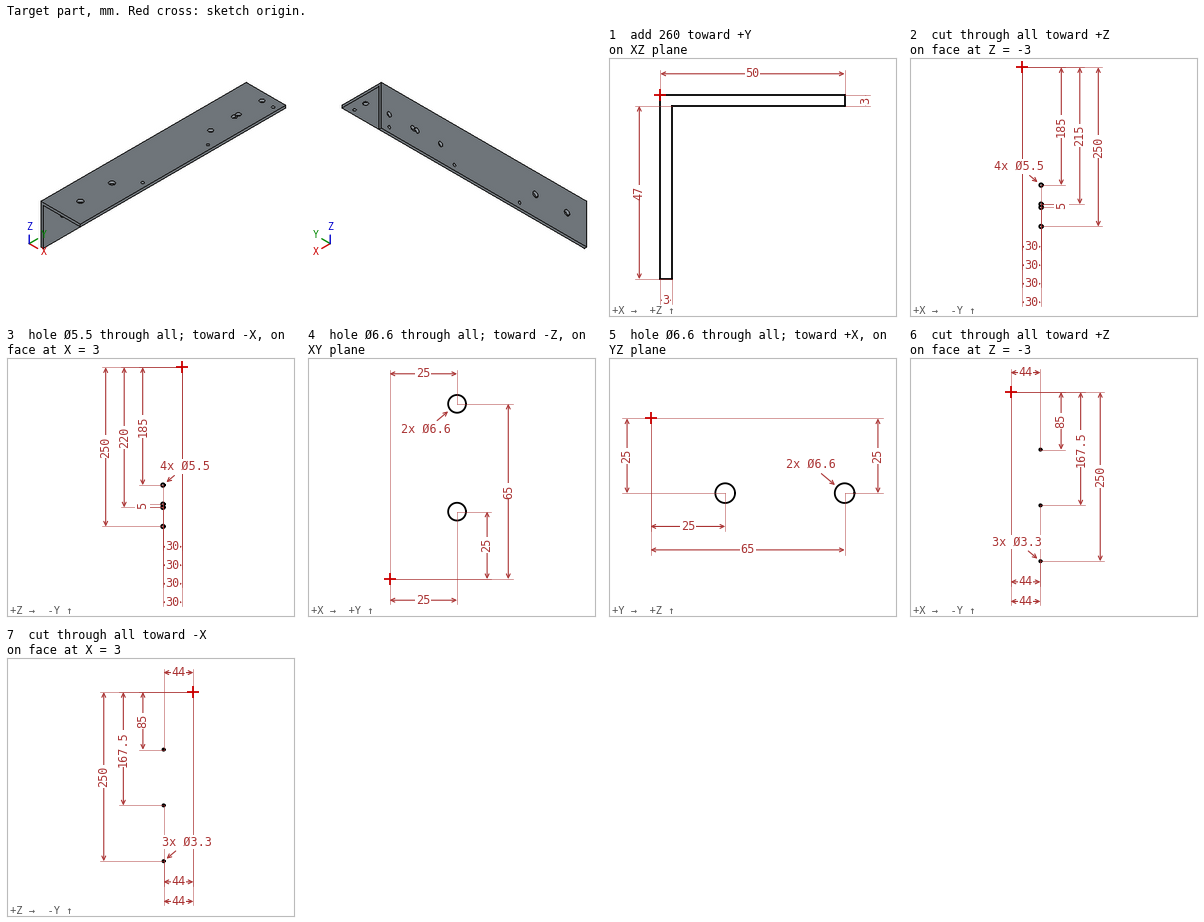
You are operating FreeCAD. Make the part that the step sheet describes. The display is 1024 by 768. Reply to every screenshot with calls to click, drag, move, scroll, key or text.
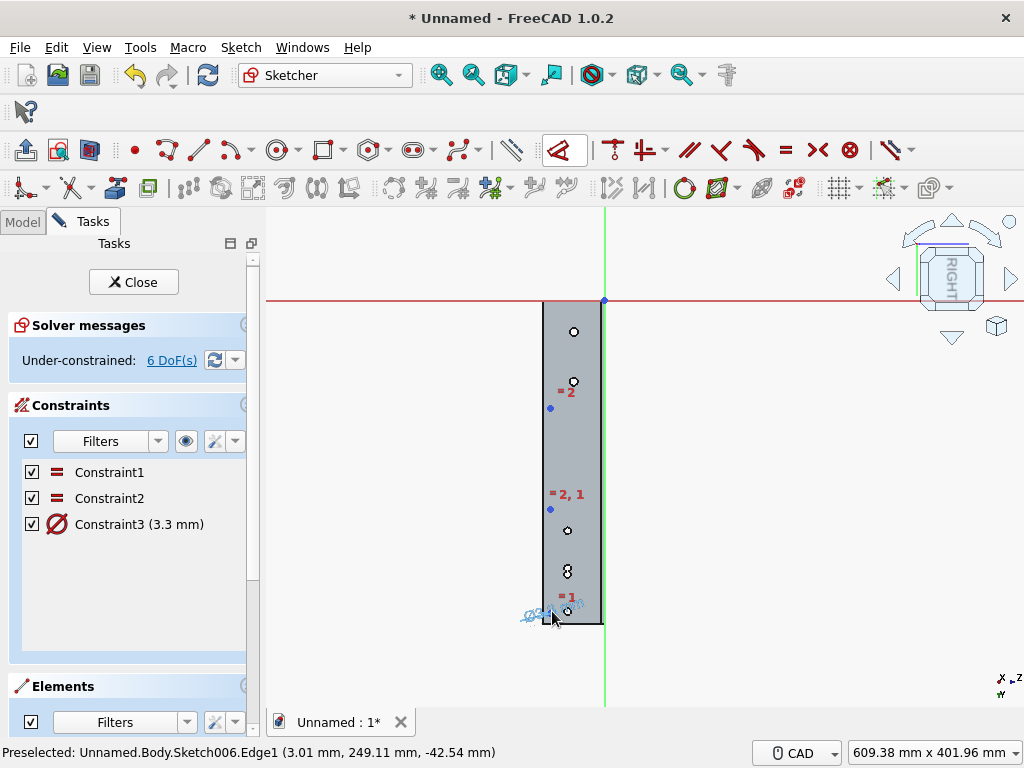
click(550, 613)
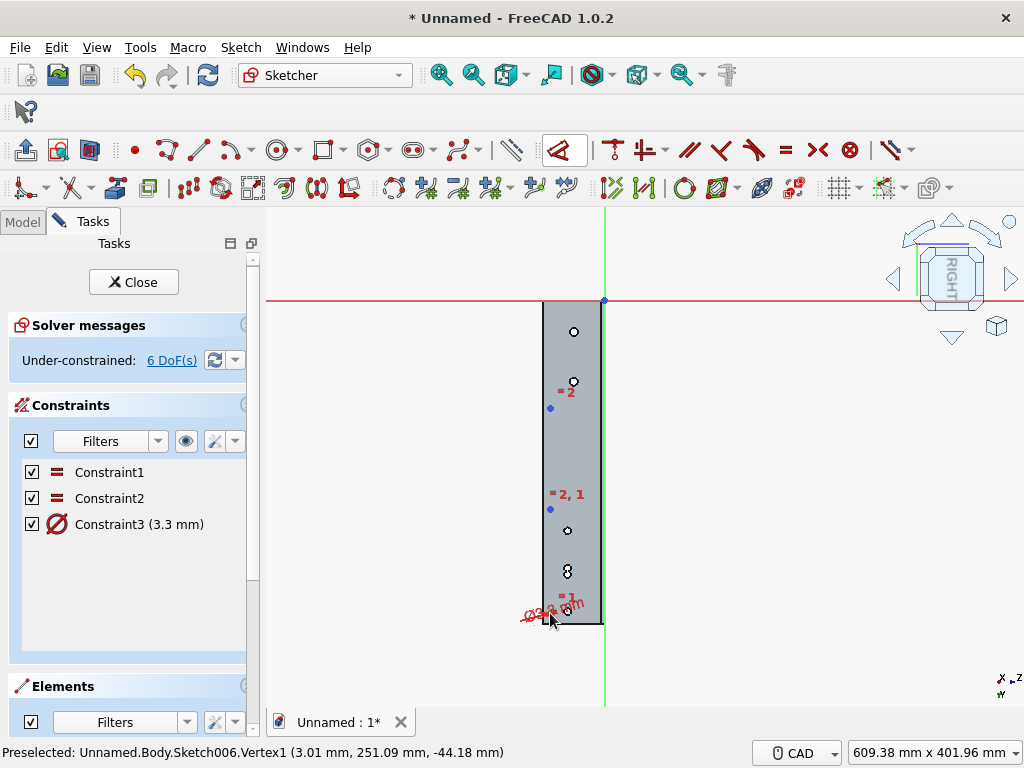
key(l)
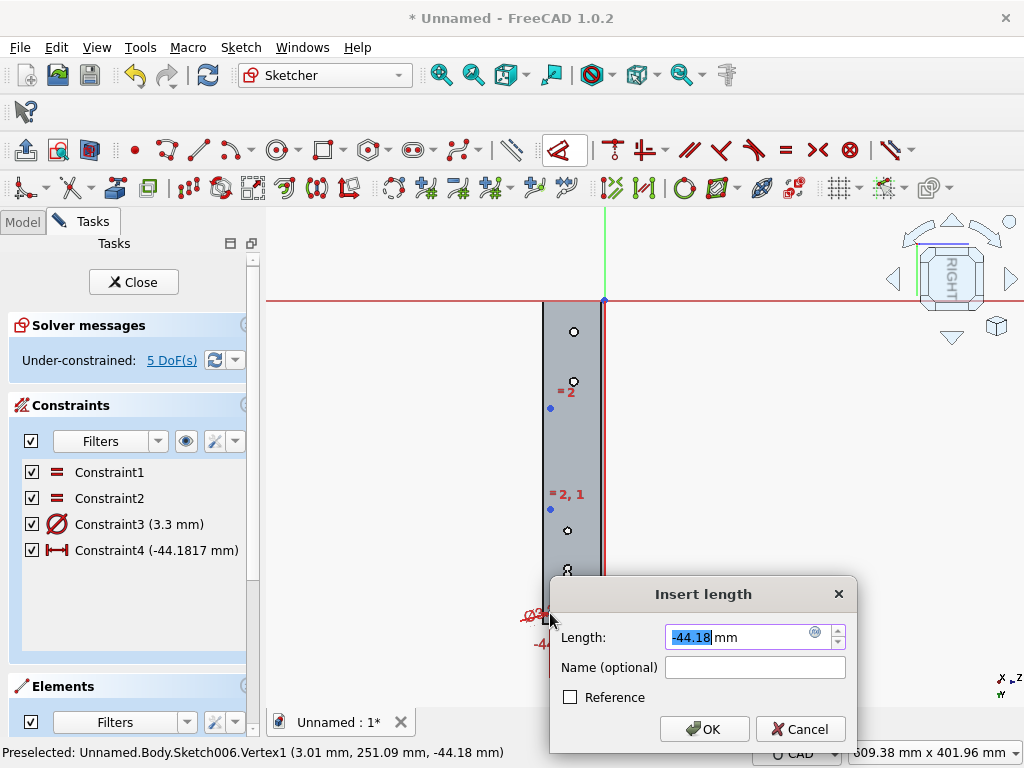
text(-44)
key(Return)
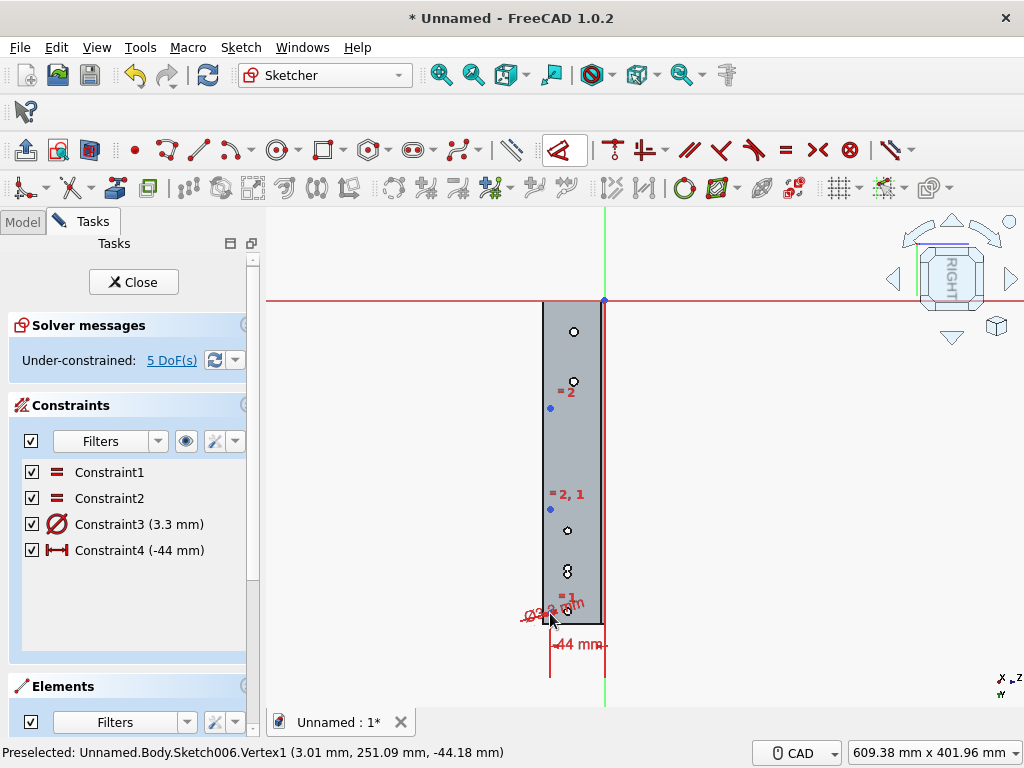
click(550, 510)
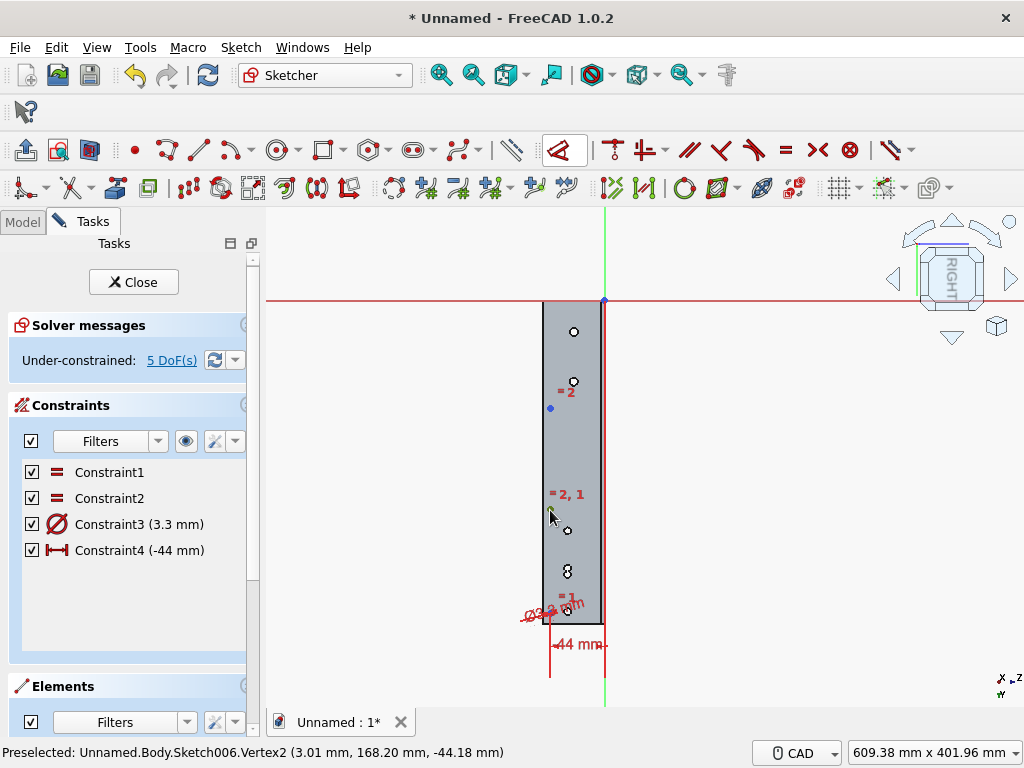
key(l)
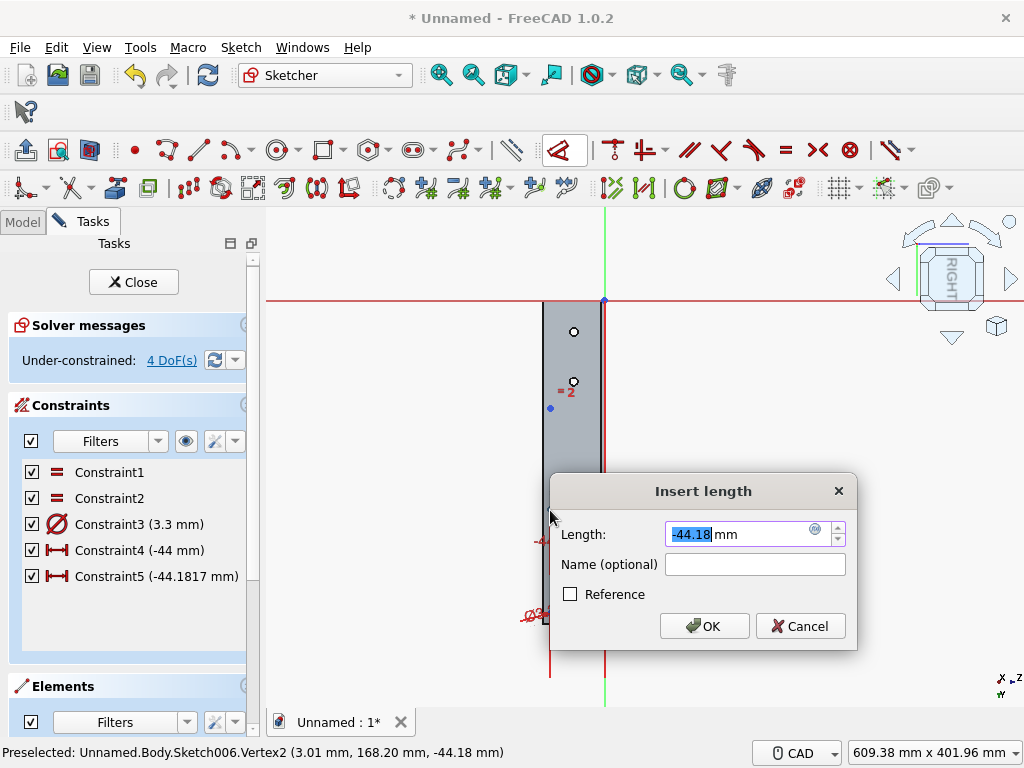
text(-44)
key(Return)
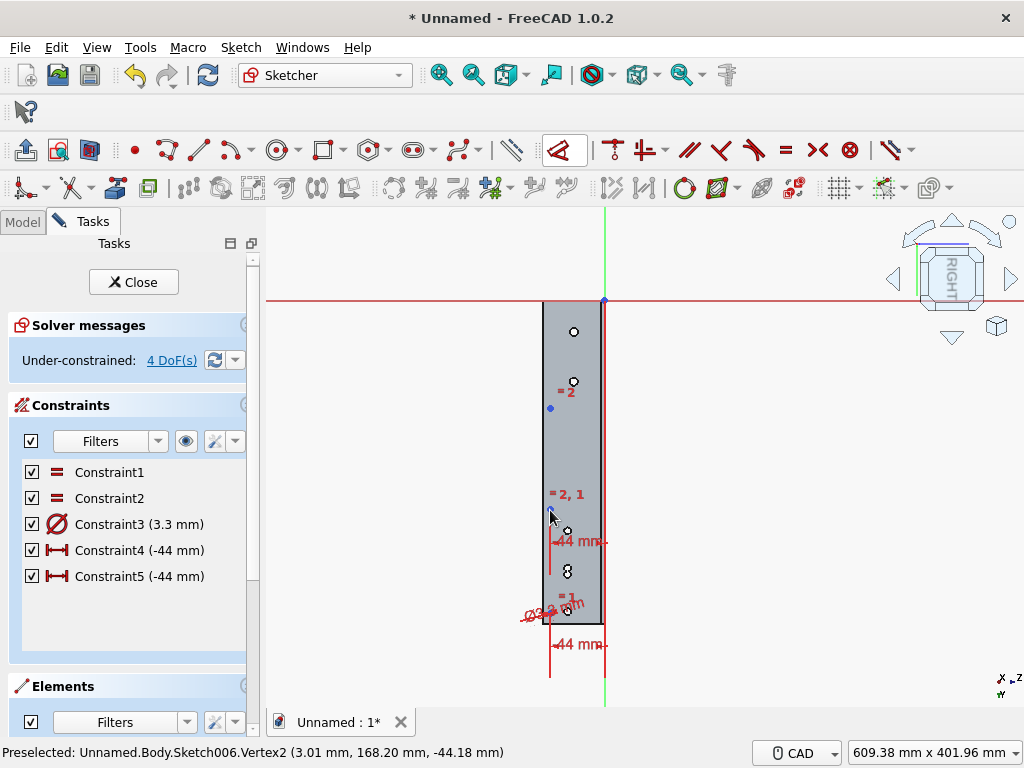
click(550, 408)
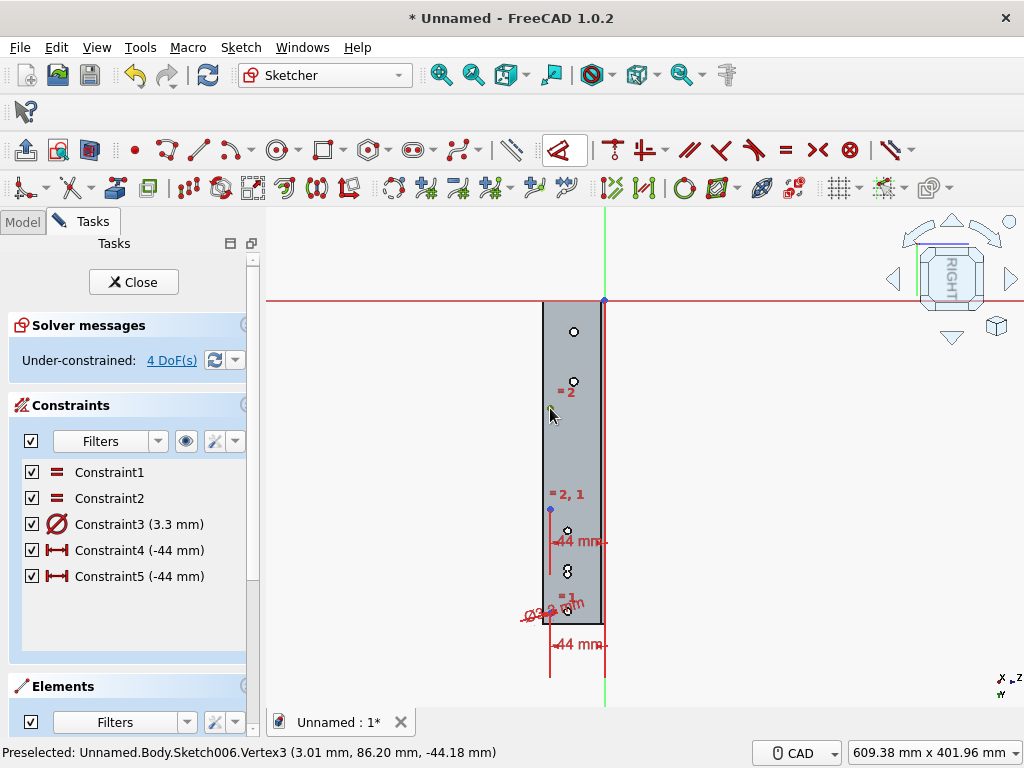
key(l)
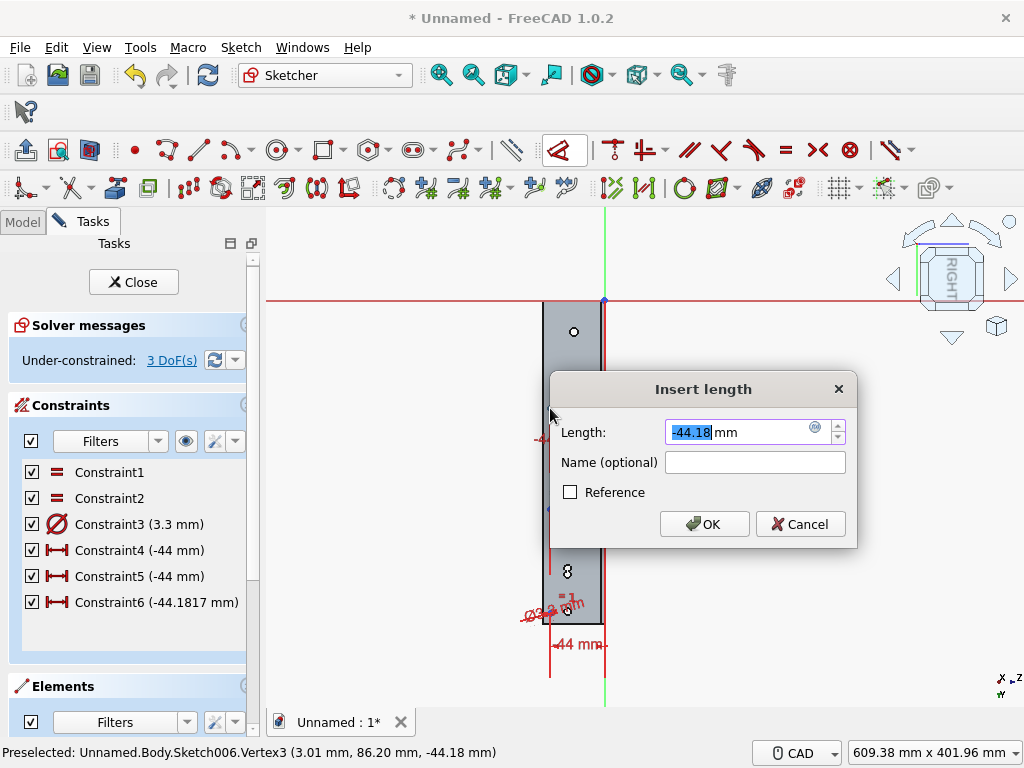
text(-44)
key(Return)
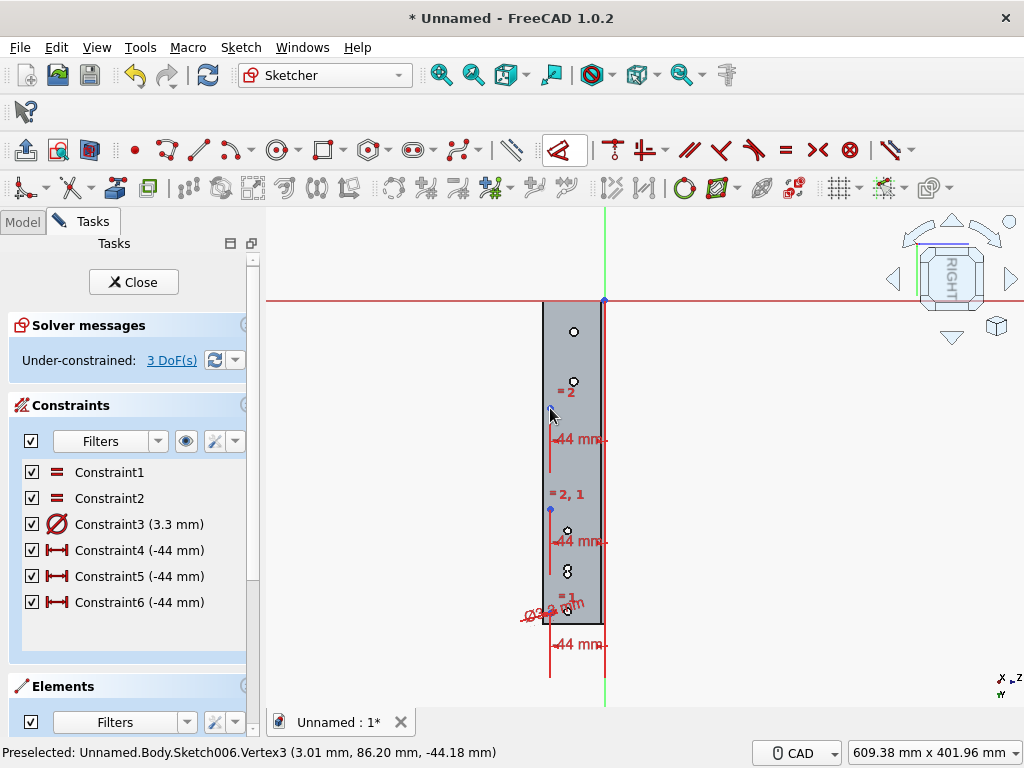
click(550, 408)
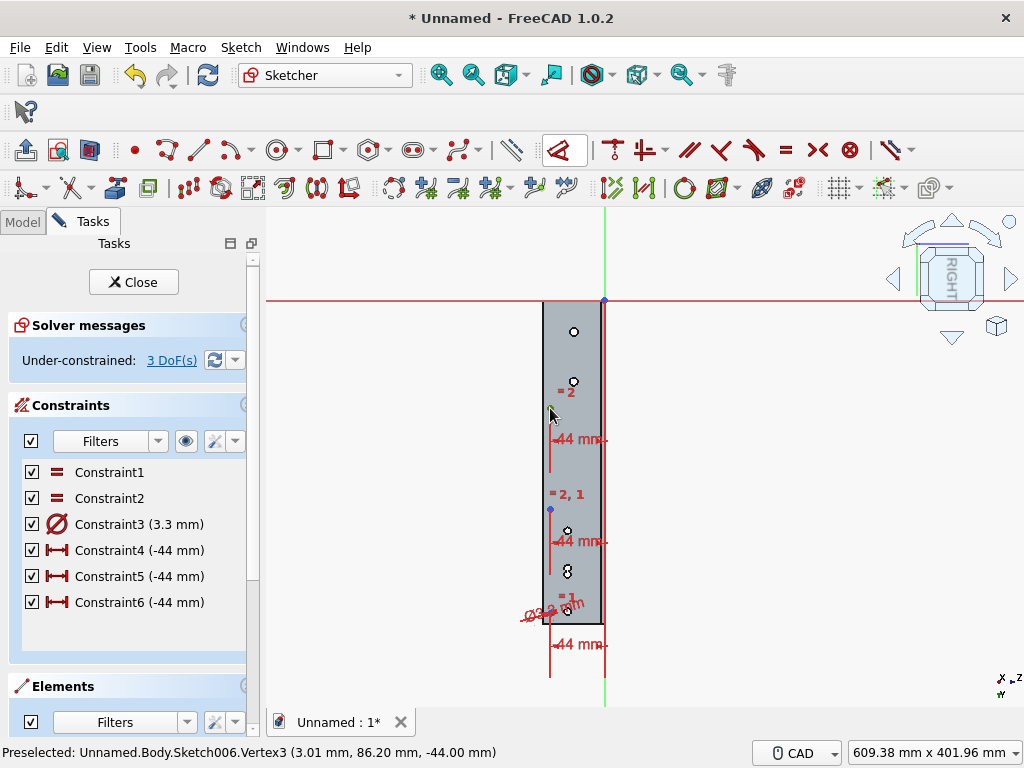
key(i)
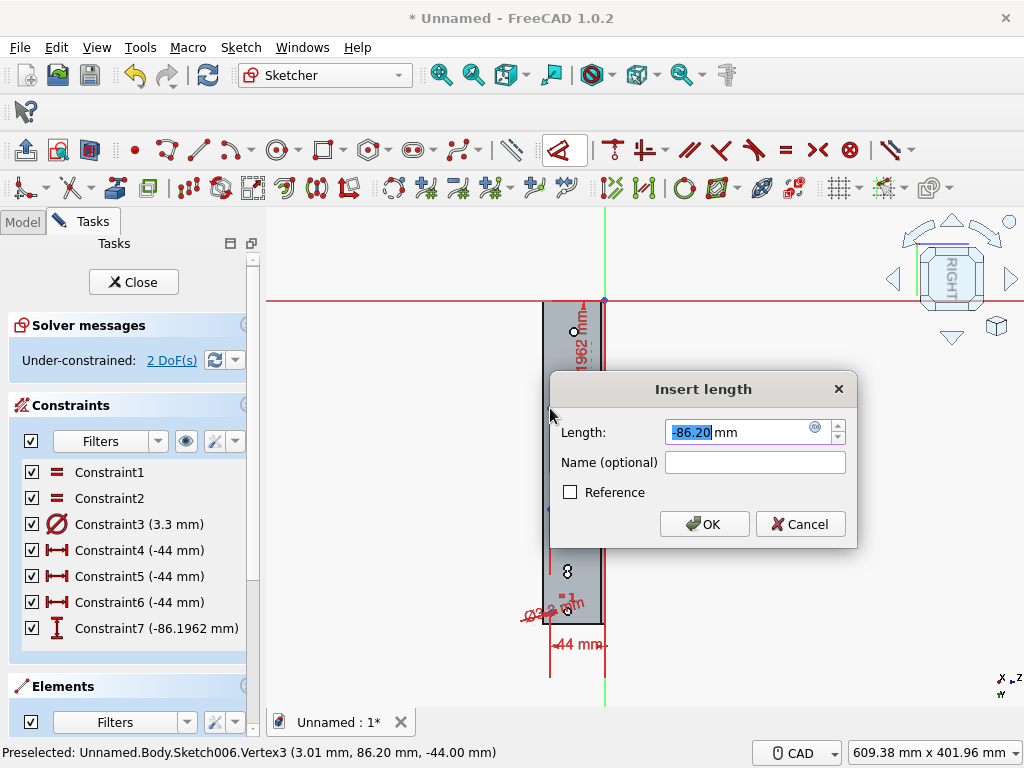
text(-85)
key(Return)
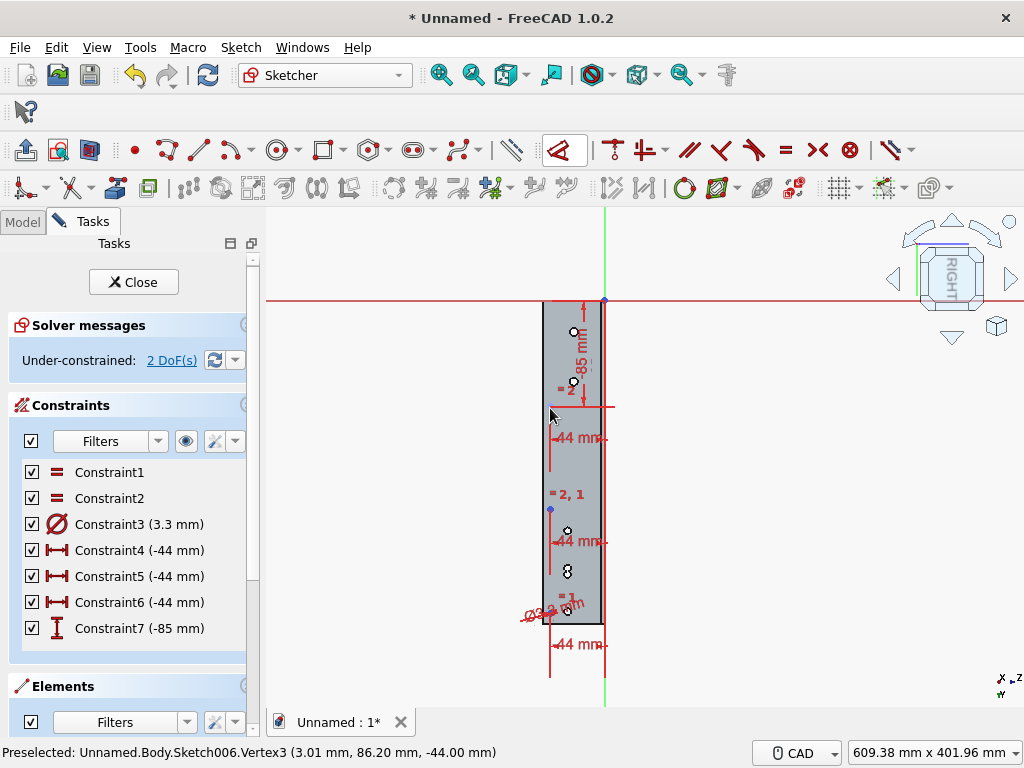
click(550, 613)